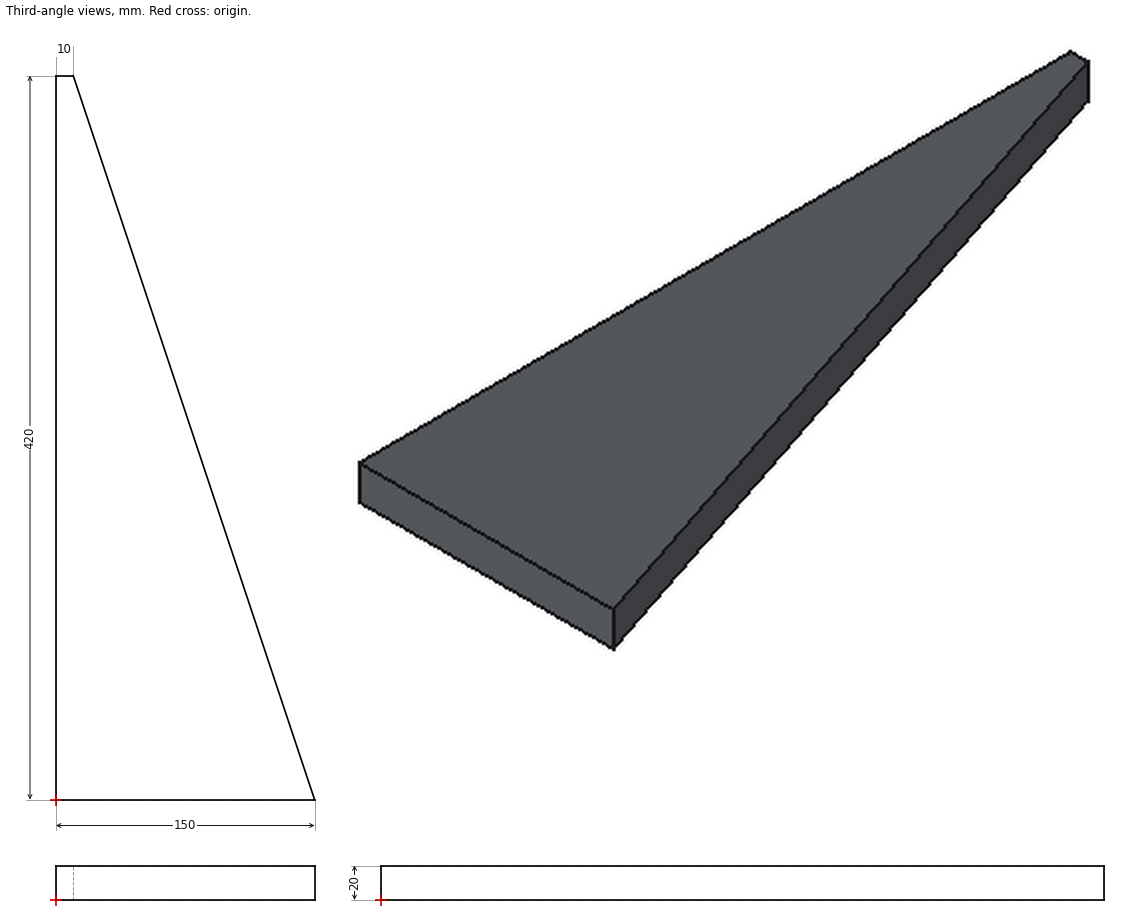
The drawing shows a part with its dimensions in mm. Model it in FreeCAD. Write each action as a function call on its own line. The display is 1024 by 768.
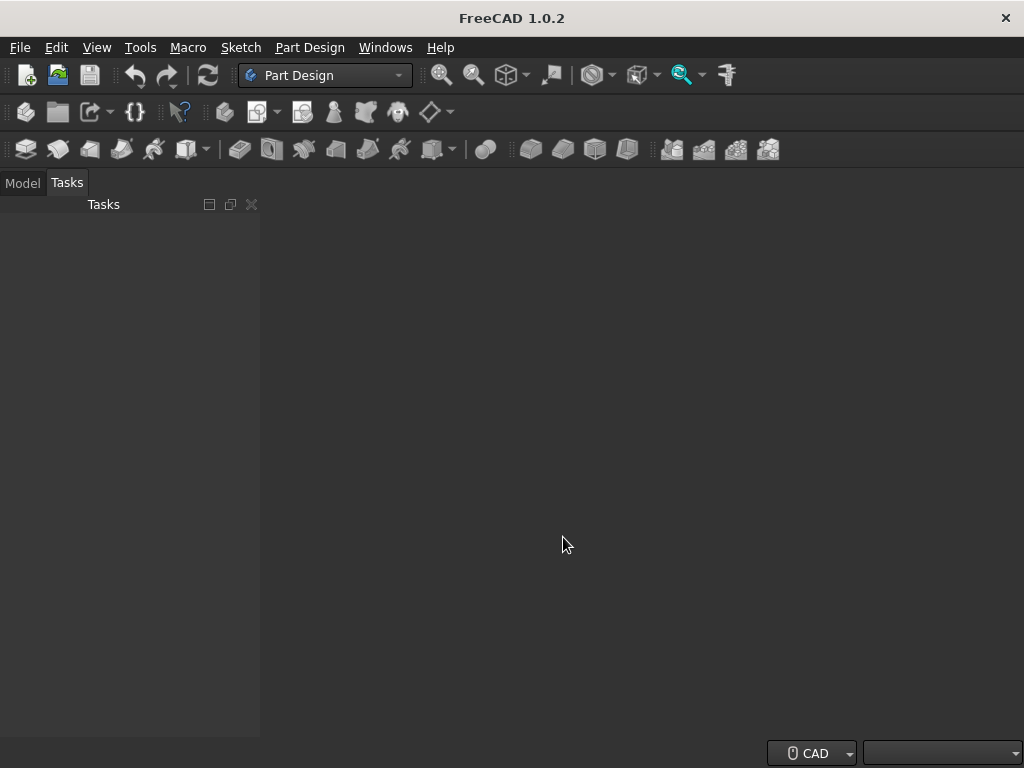
click(26, 76)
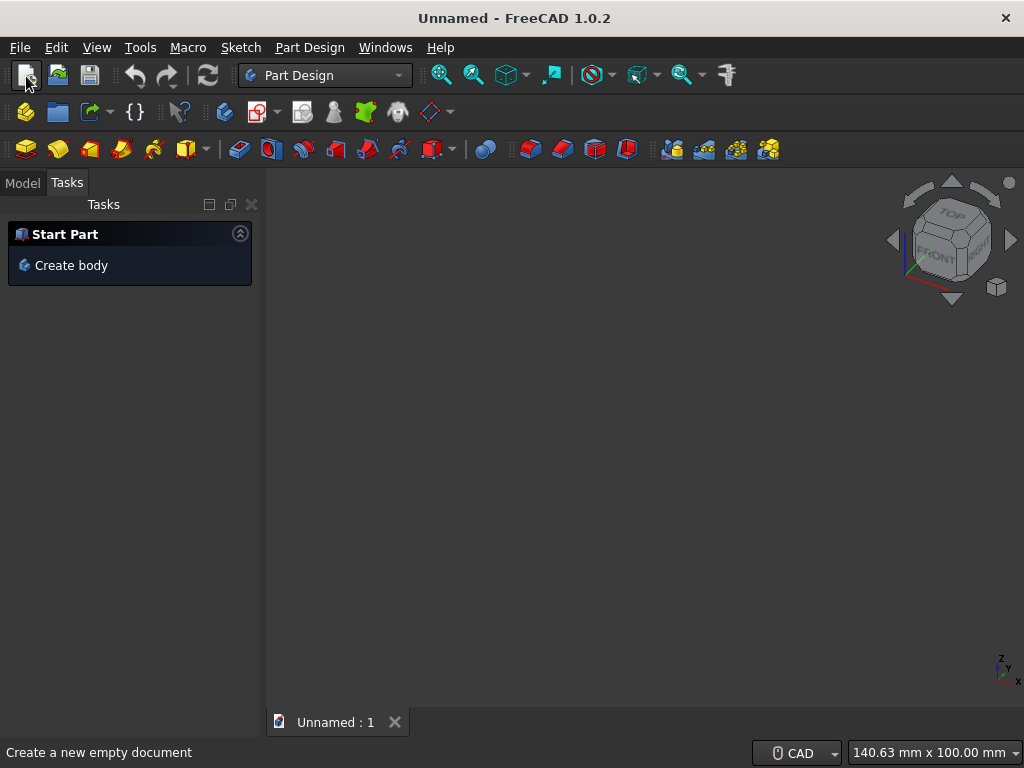
click(258, 112)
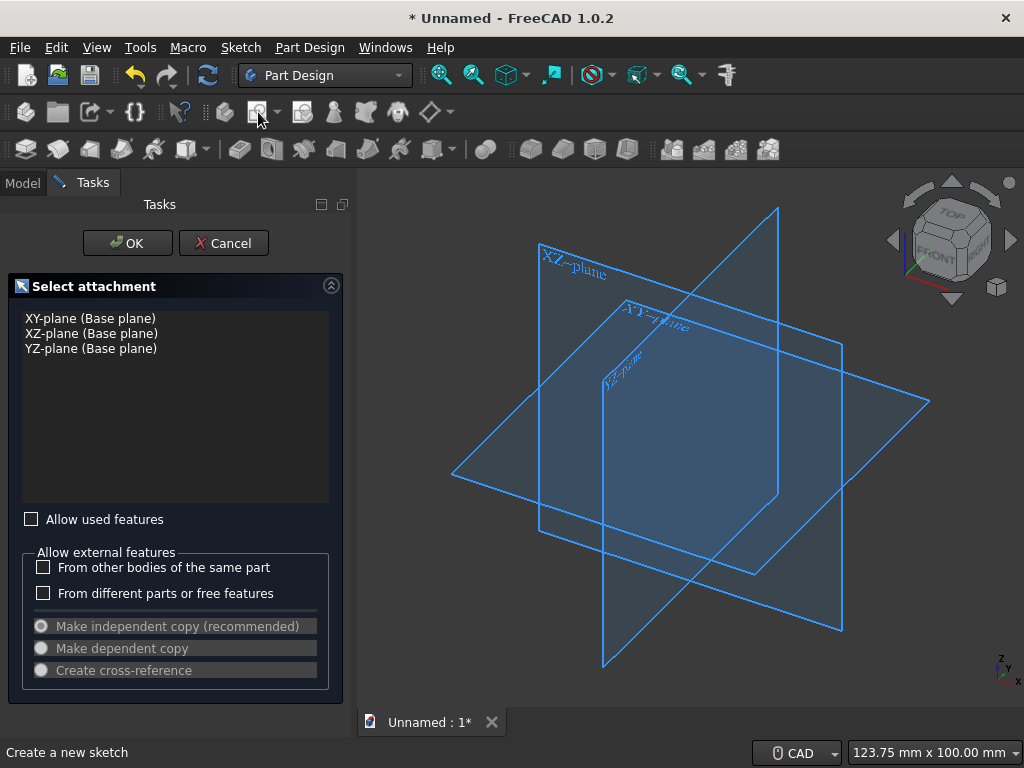
click(82, 318)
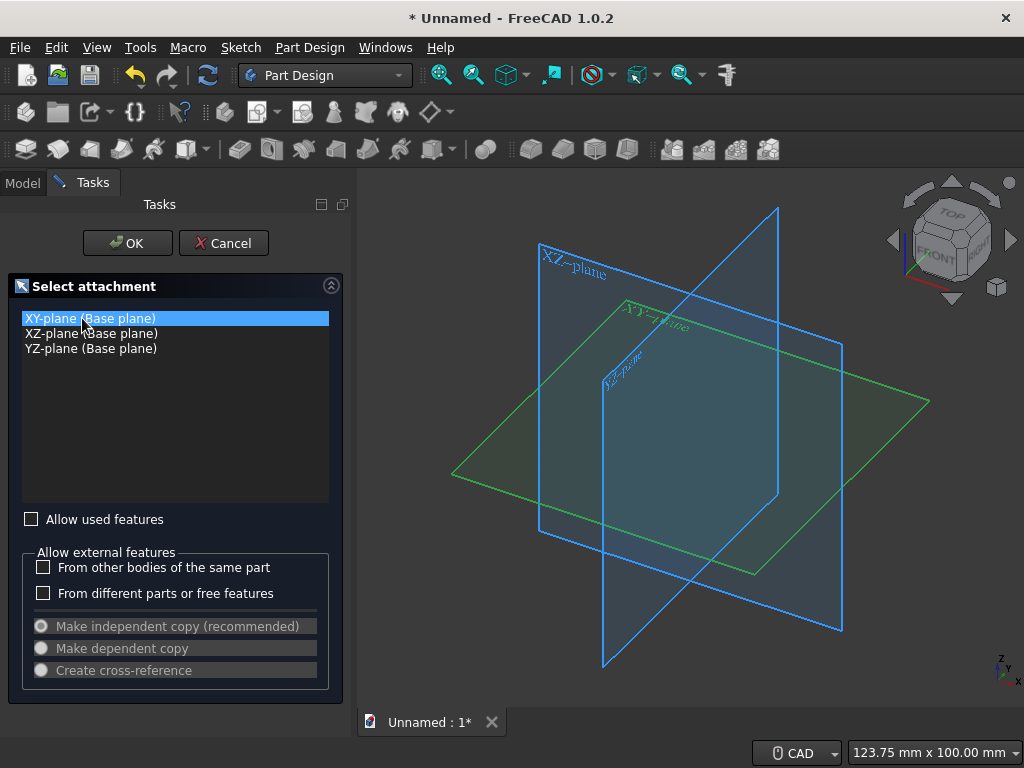
click(128, 243)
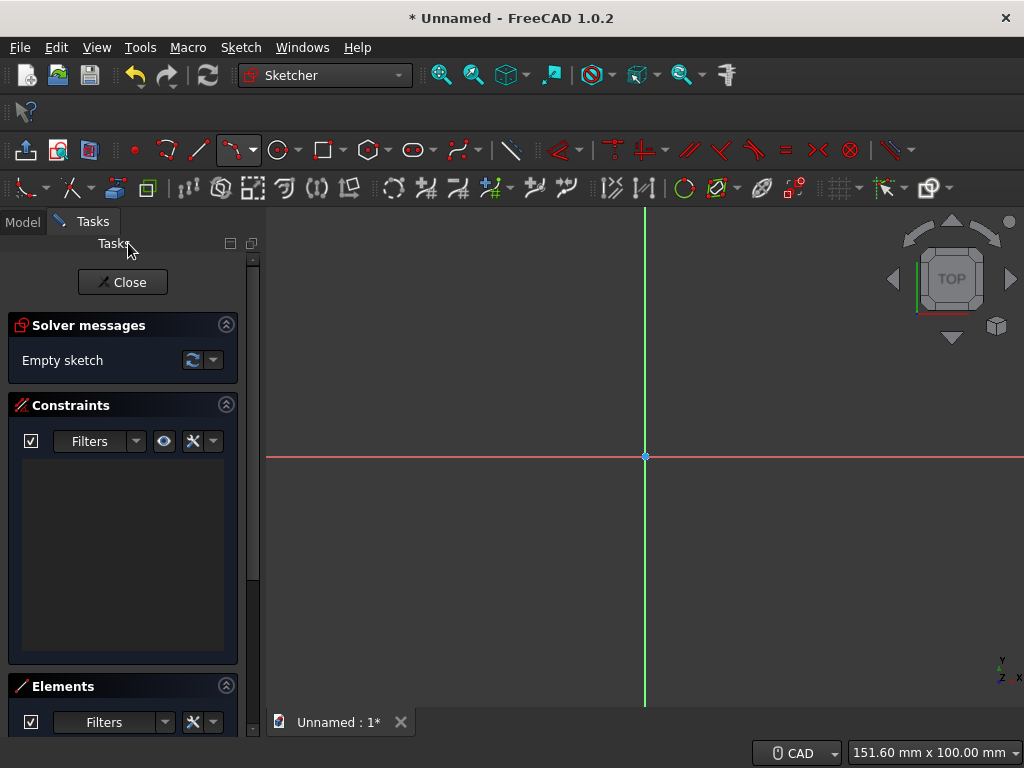
scroll(507, 621, down, 10)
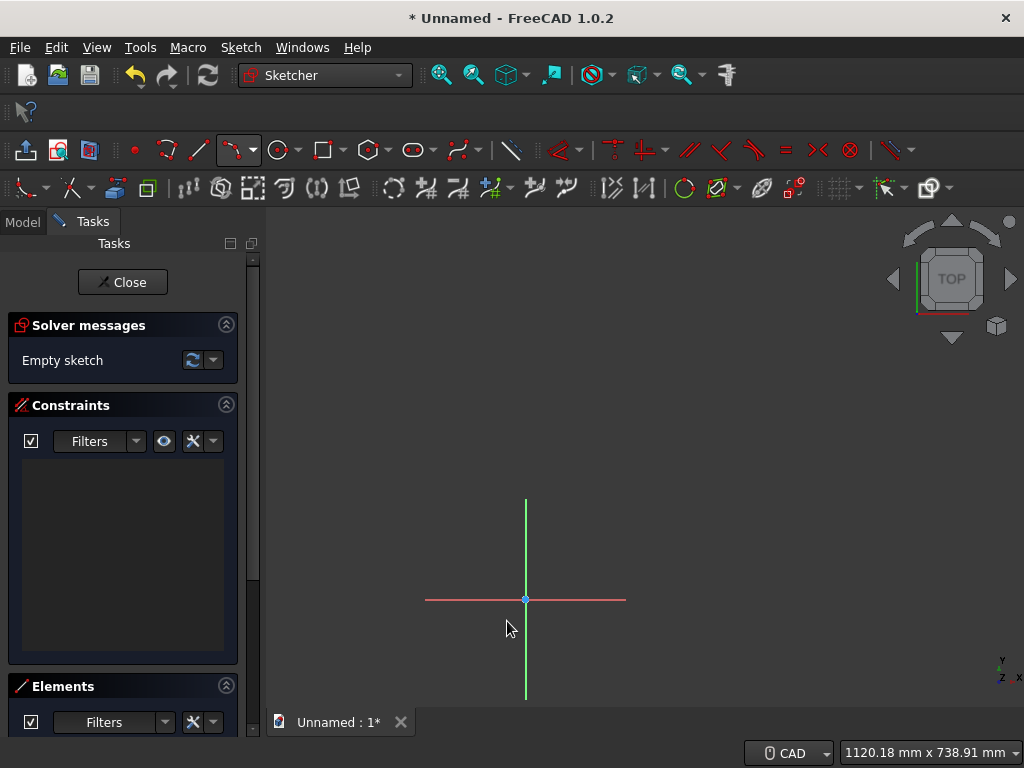
key(g)
key(m)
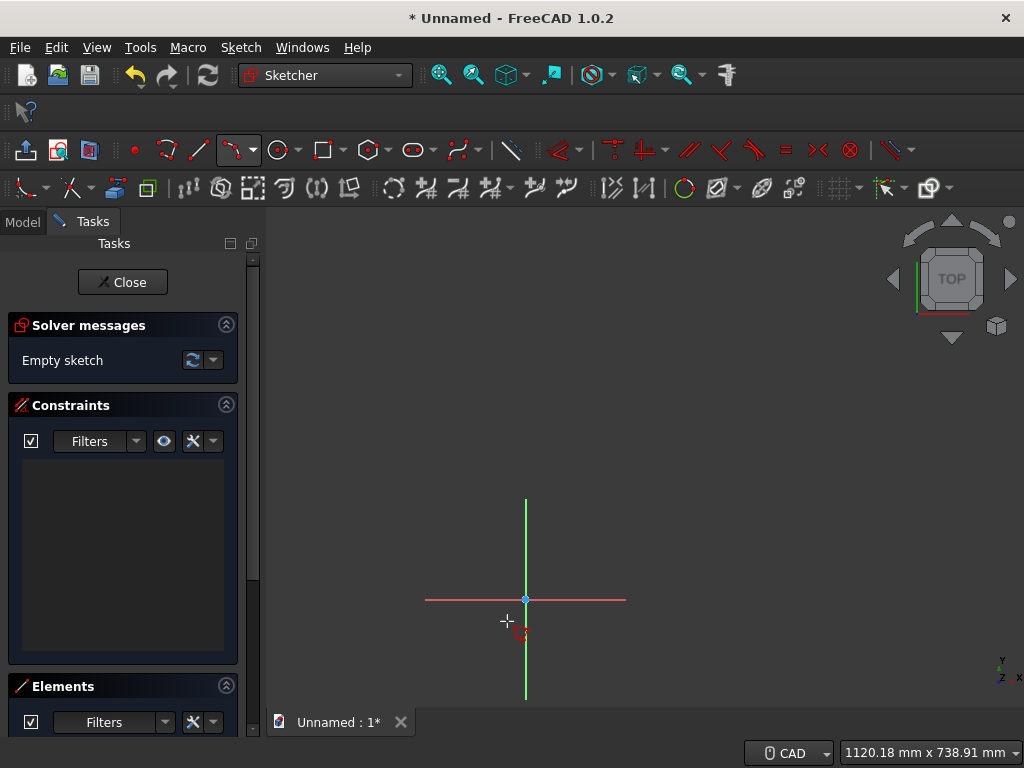
click(526, 600)
click(627, 591)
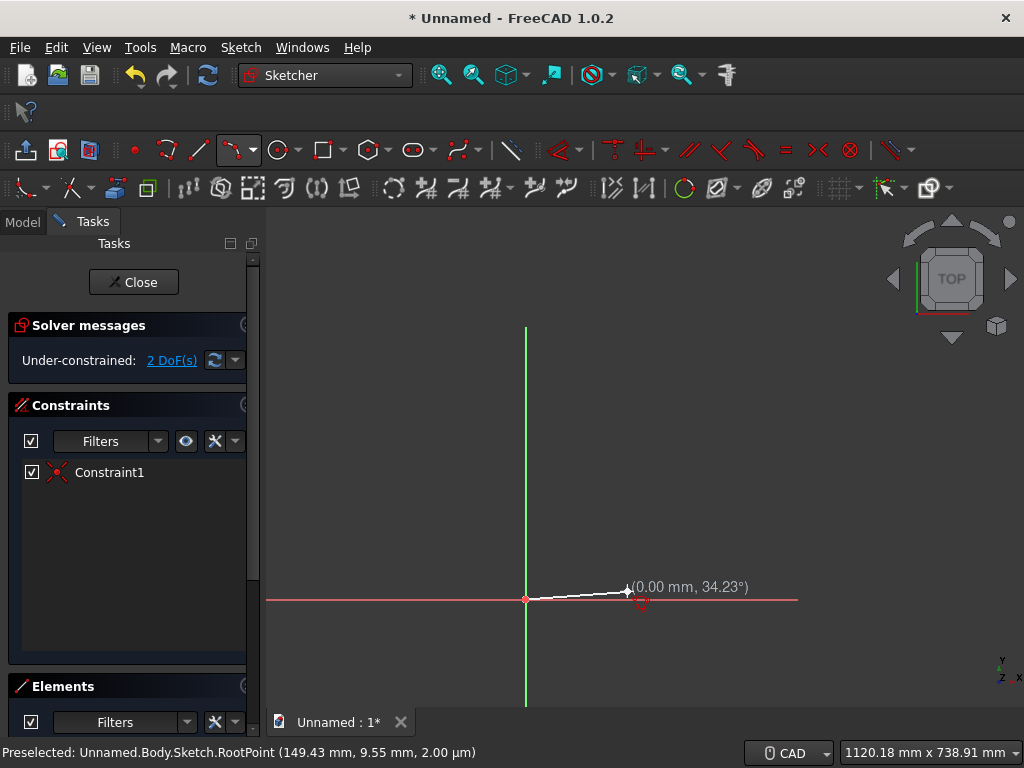
scroll(533, 315, up, 5)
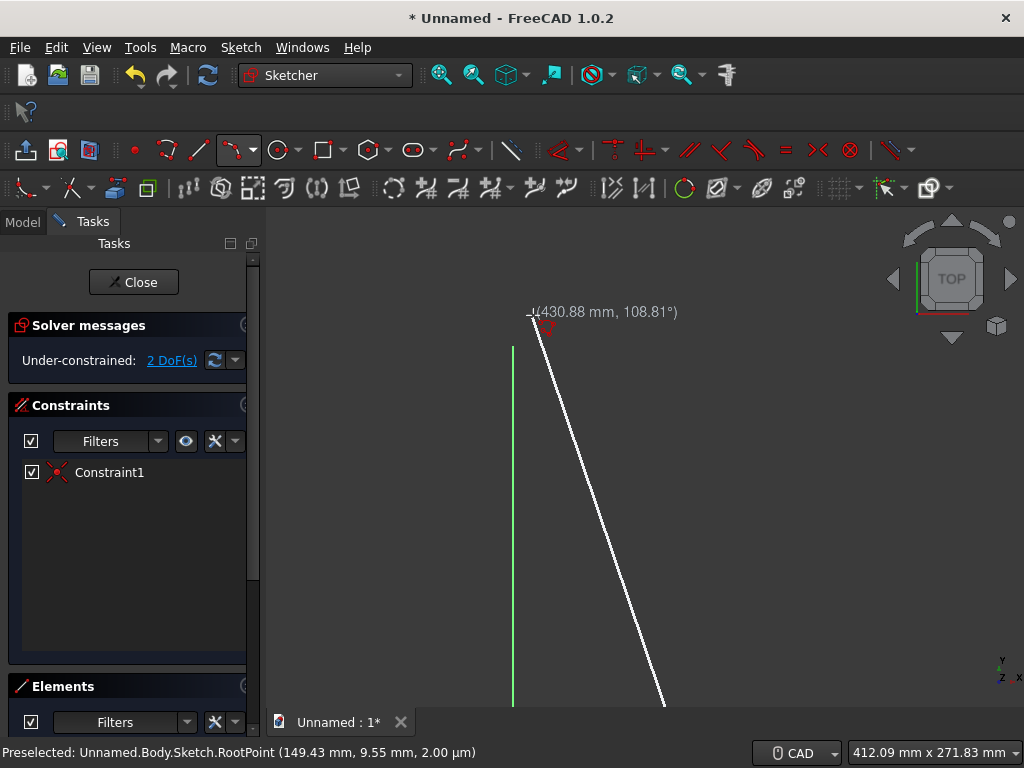
click(532, 315)
click(522, 315)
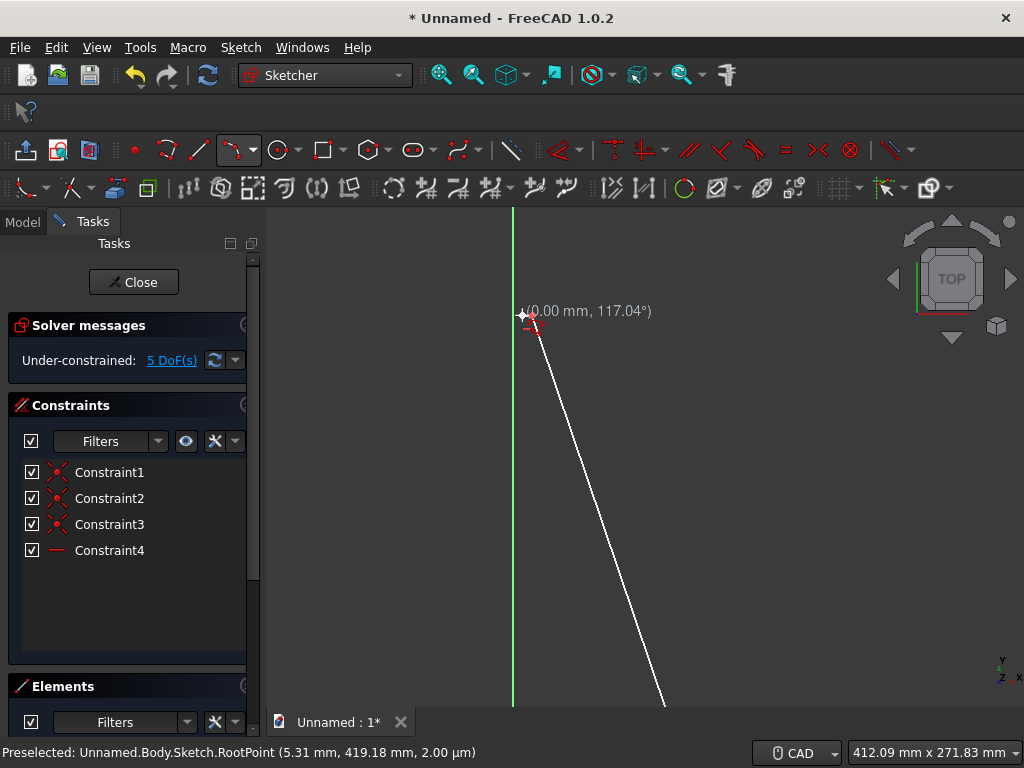
scroll(533, 315, down, 5)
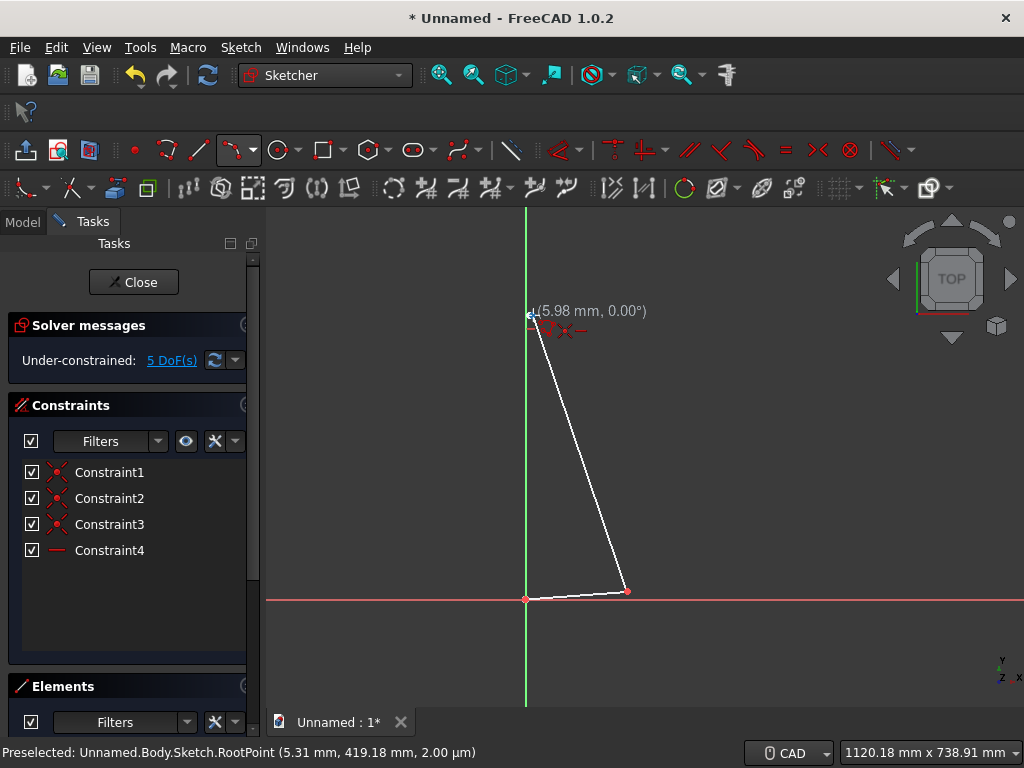
click(526, 600)
key(Escape)
key(Escape)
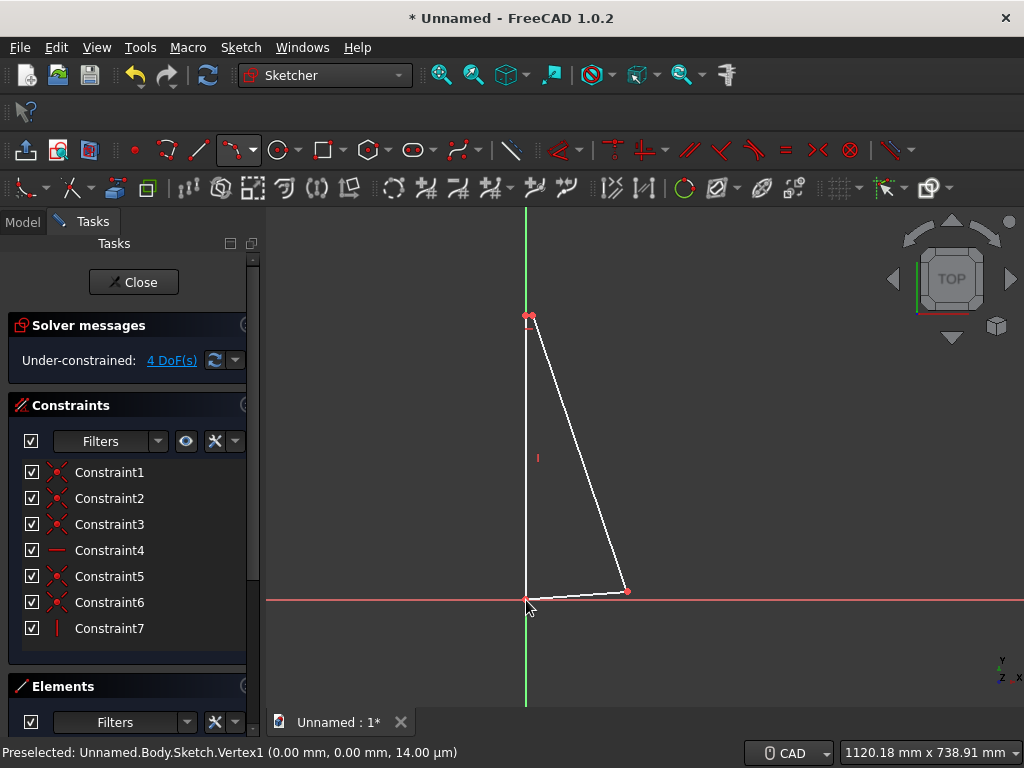
click(556, 597)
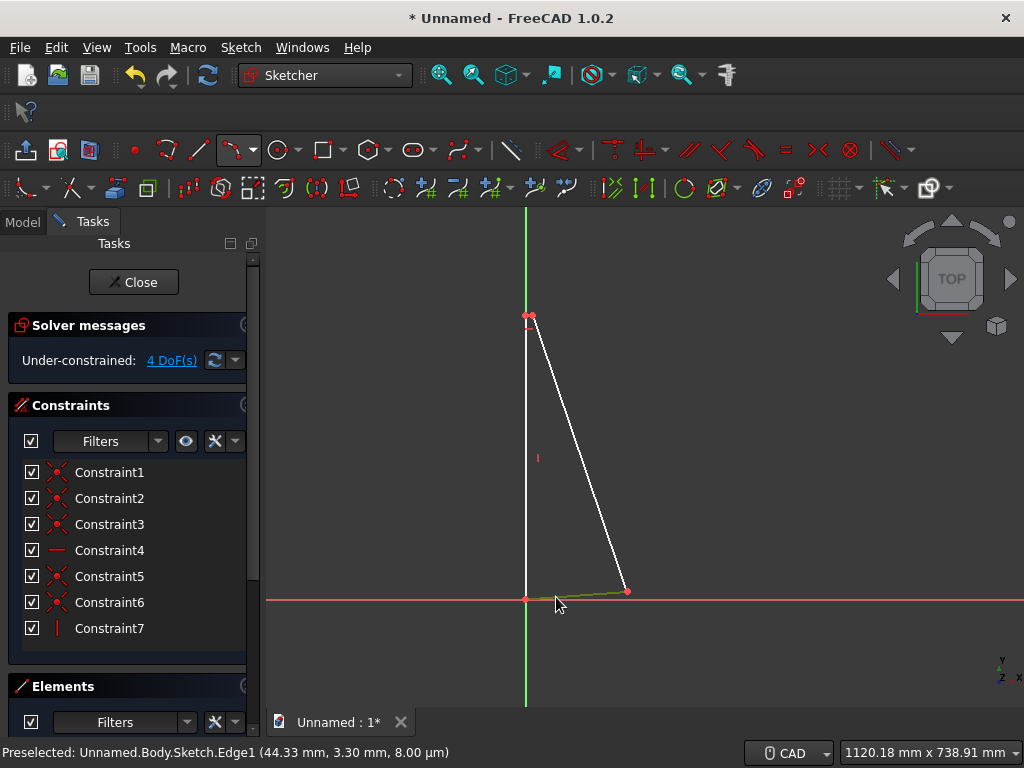
click(668, 150)